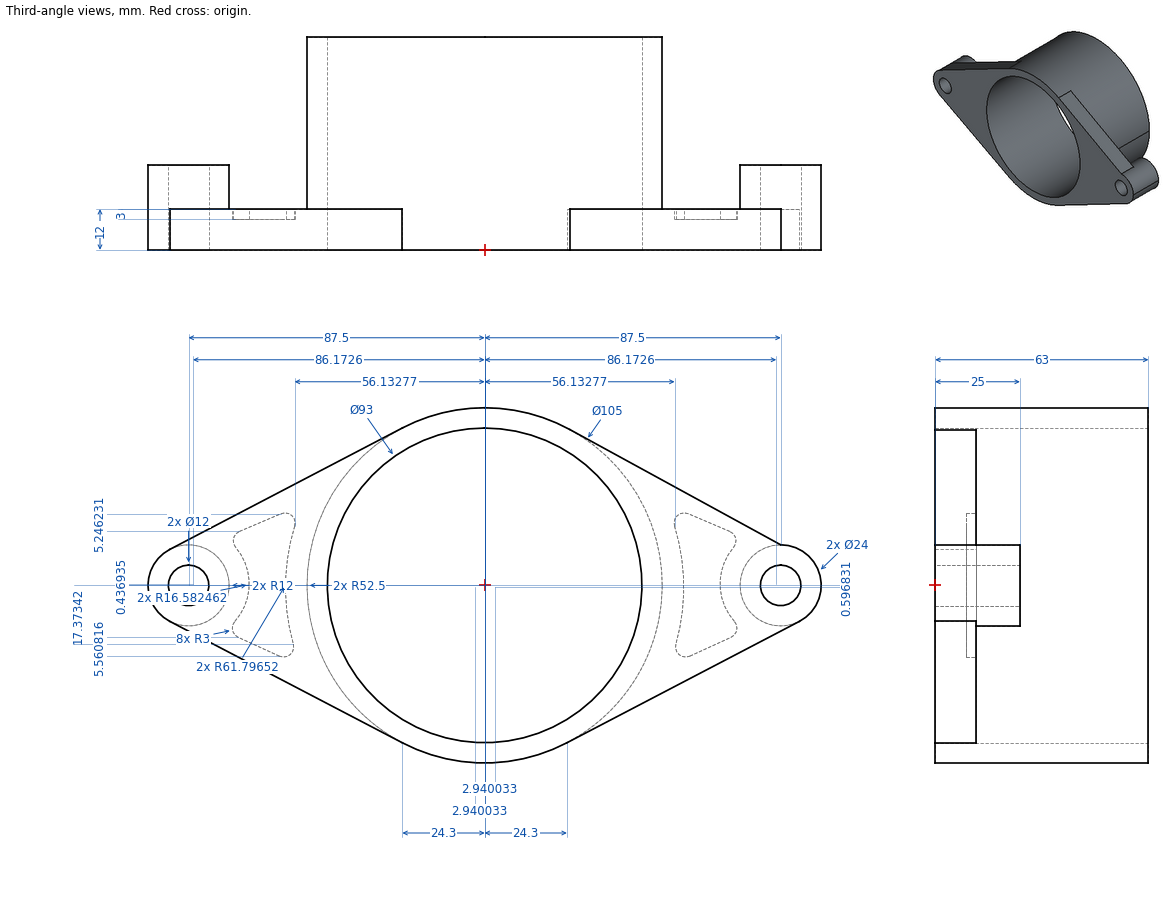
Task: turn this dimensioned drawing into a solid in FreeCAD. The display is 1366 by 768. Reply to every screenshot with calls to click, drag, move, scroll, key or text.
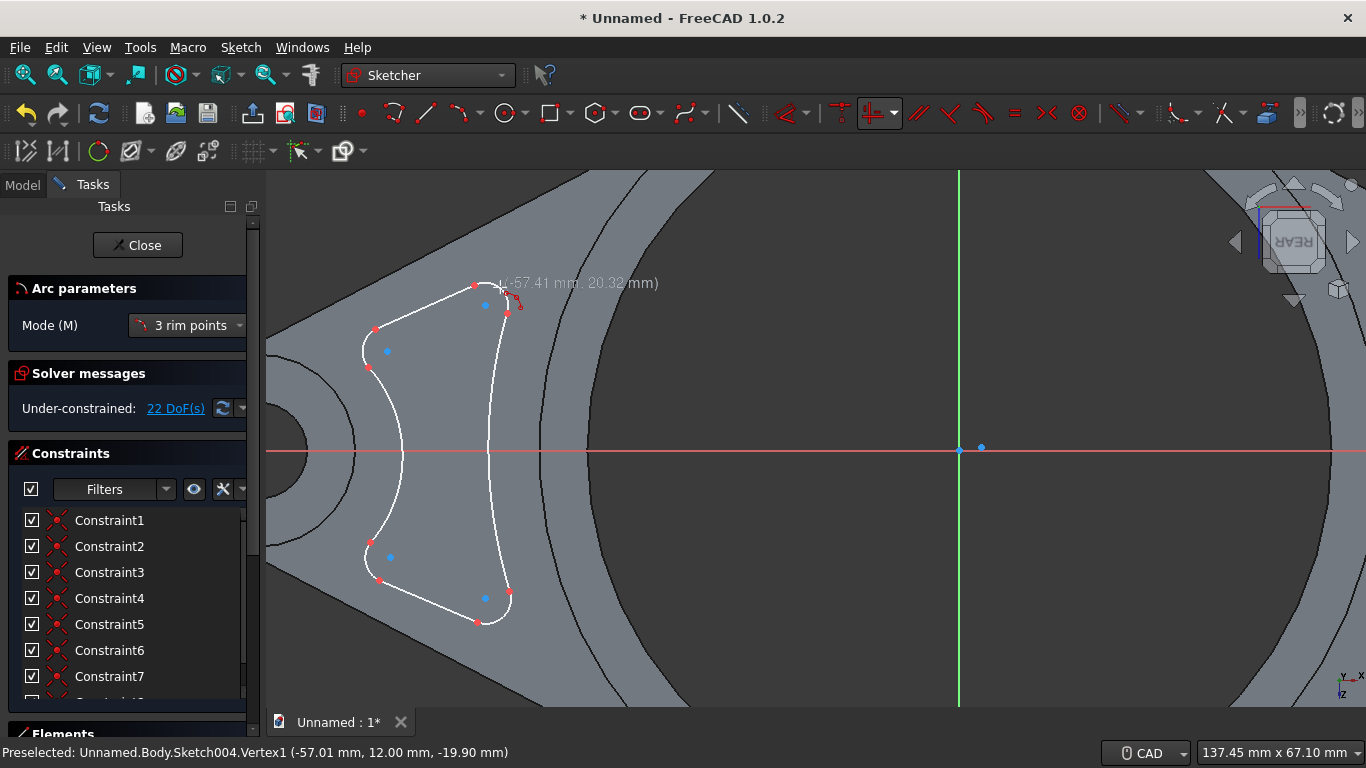
key(g)
key(l)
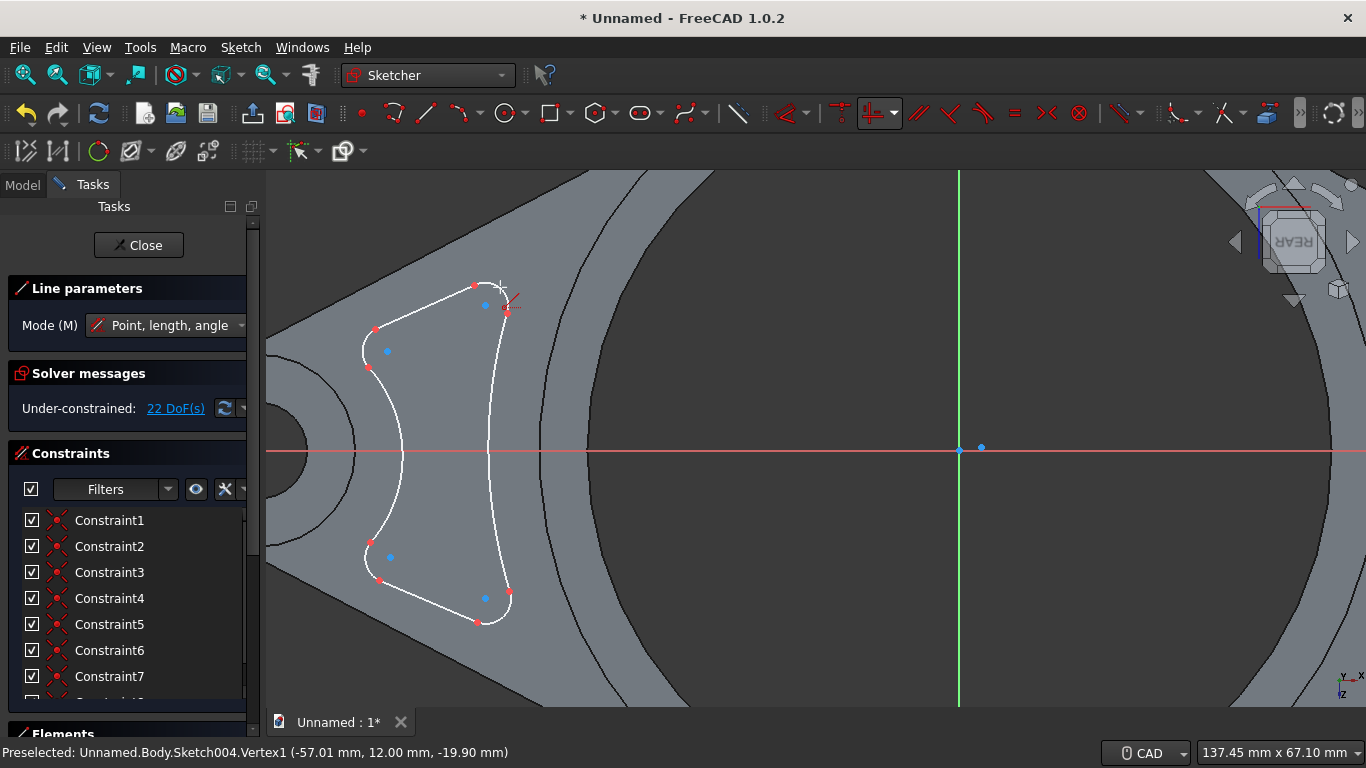
scroll(490, 422, down, 3)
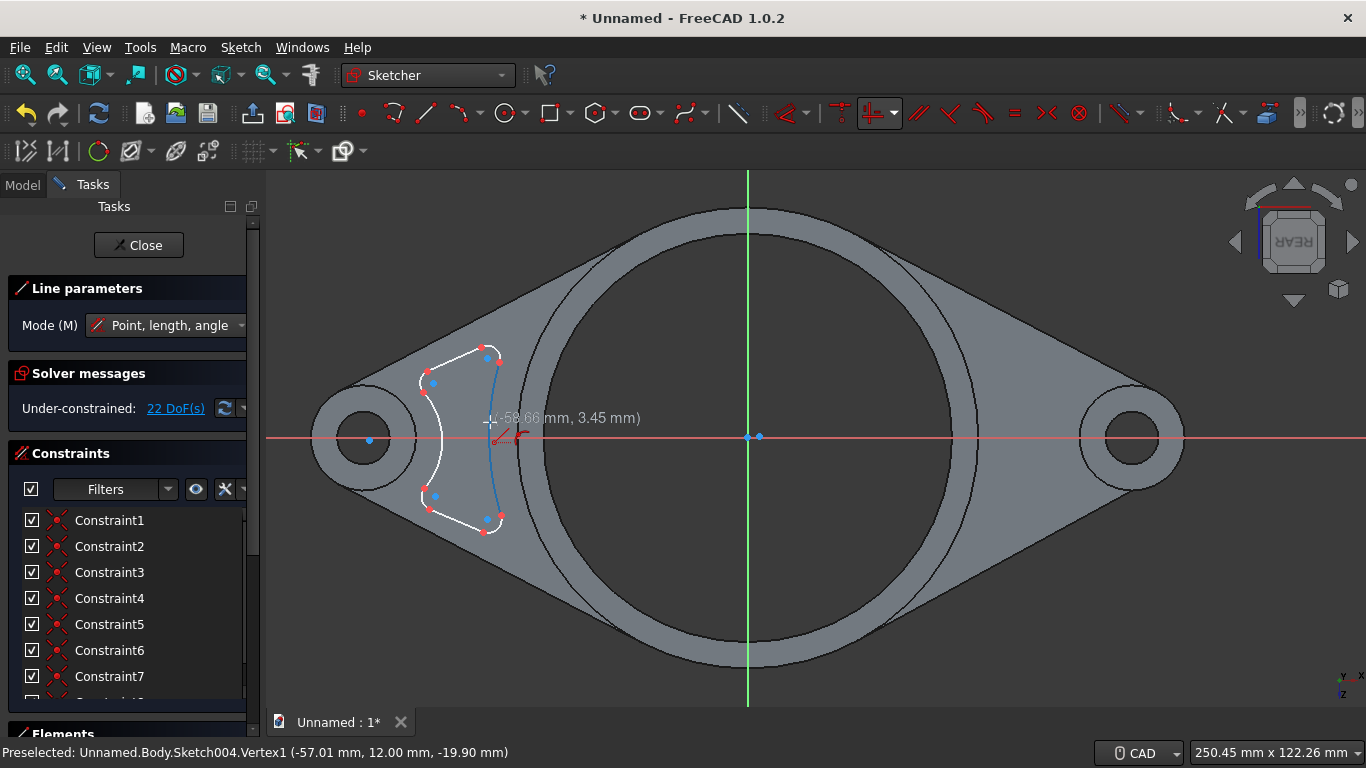
click(1068, 370)
click(1014, 346)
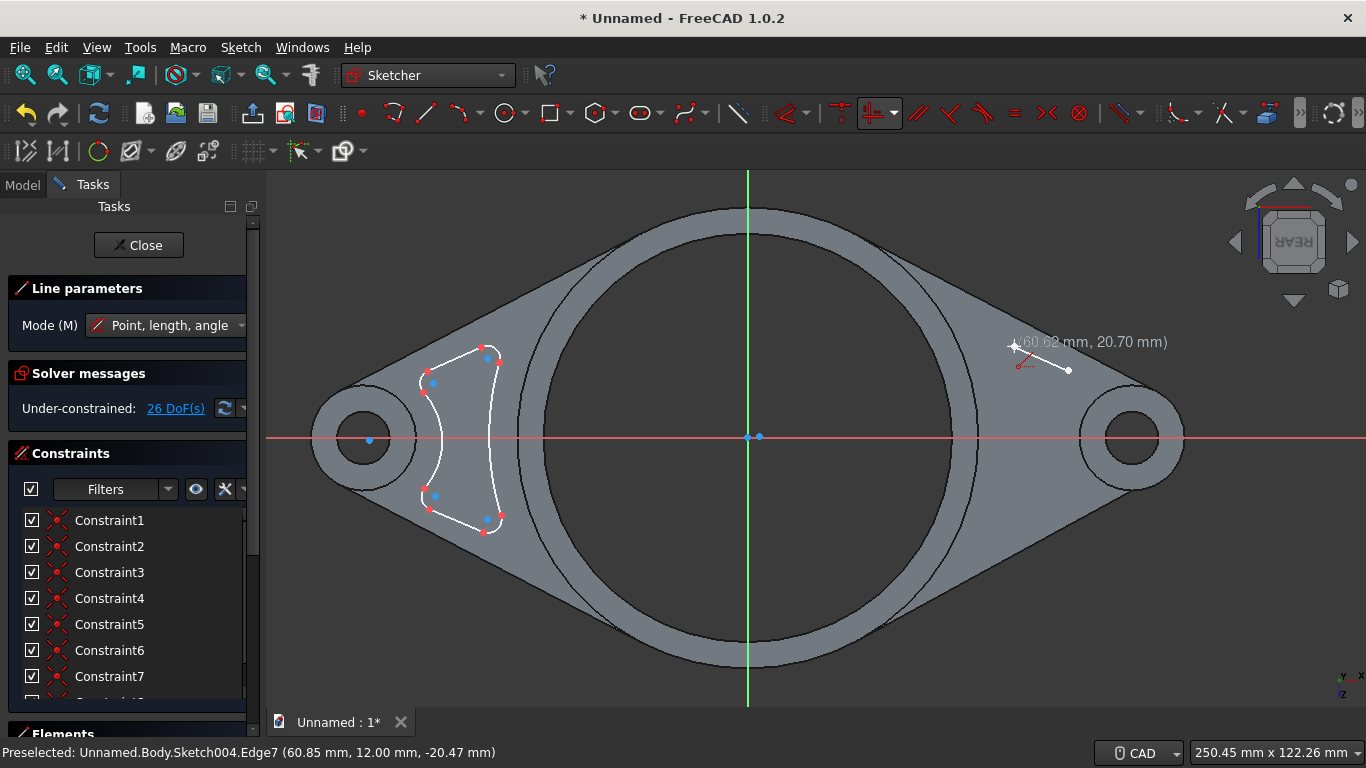
click(1012, 531)
click(1066, 508)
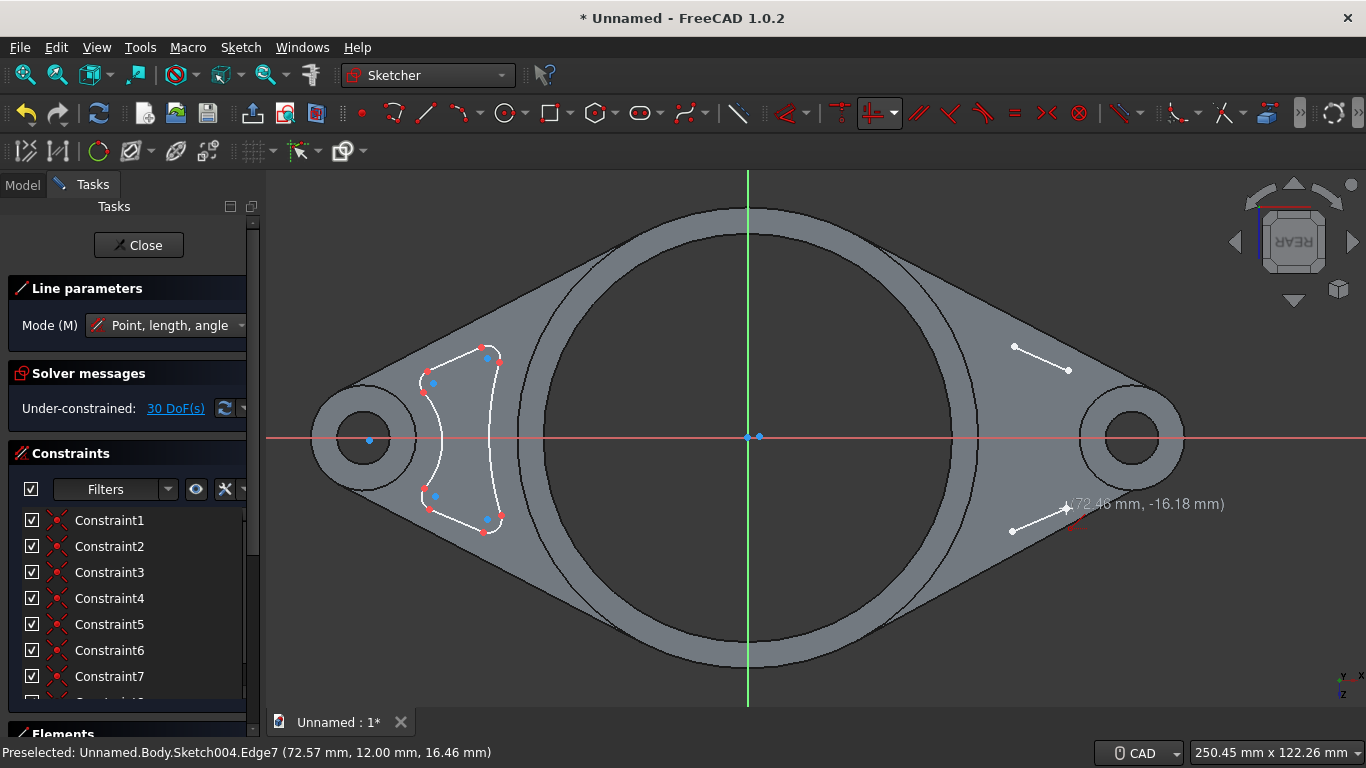
click(460, 114)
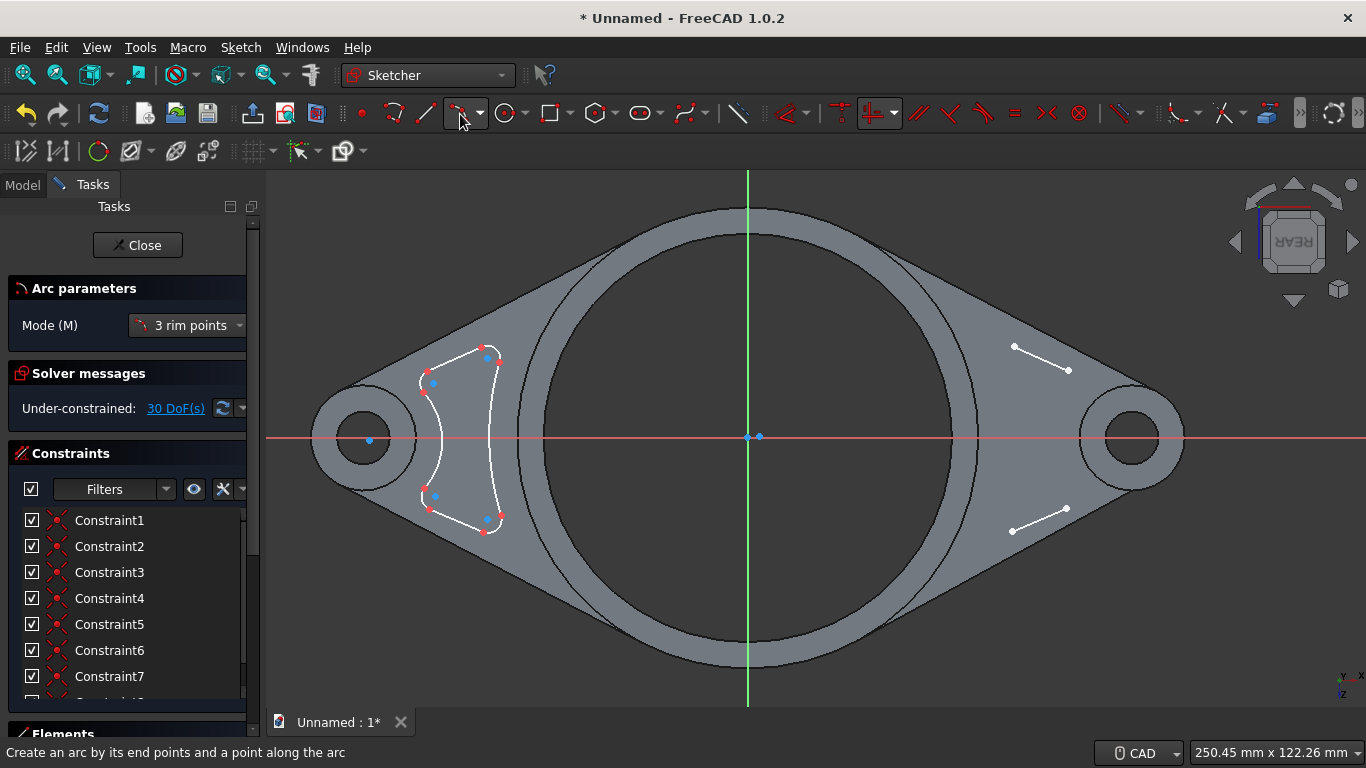
click(1014, 347)
click(996, 362)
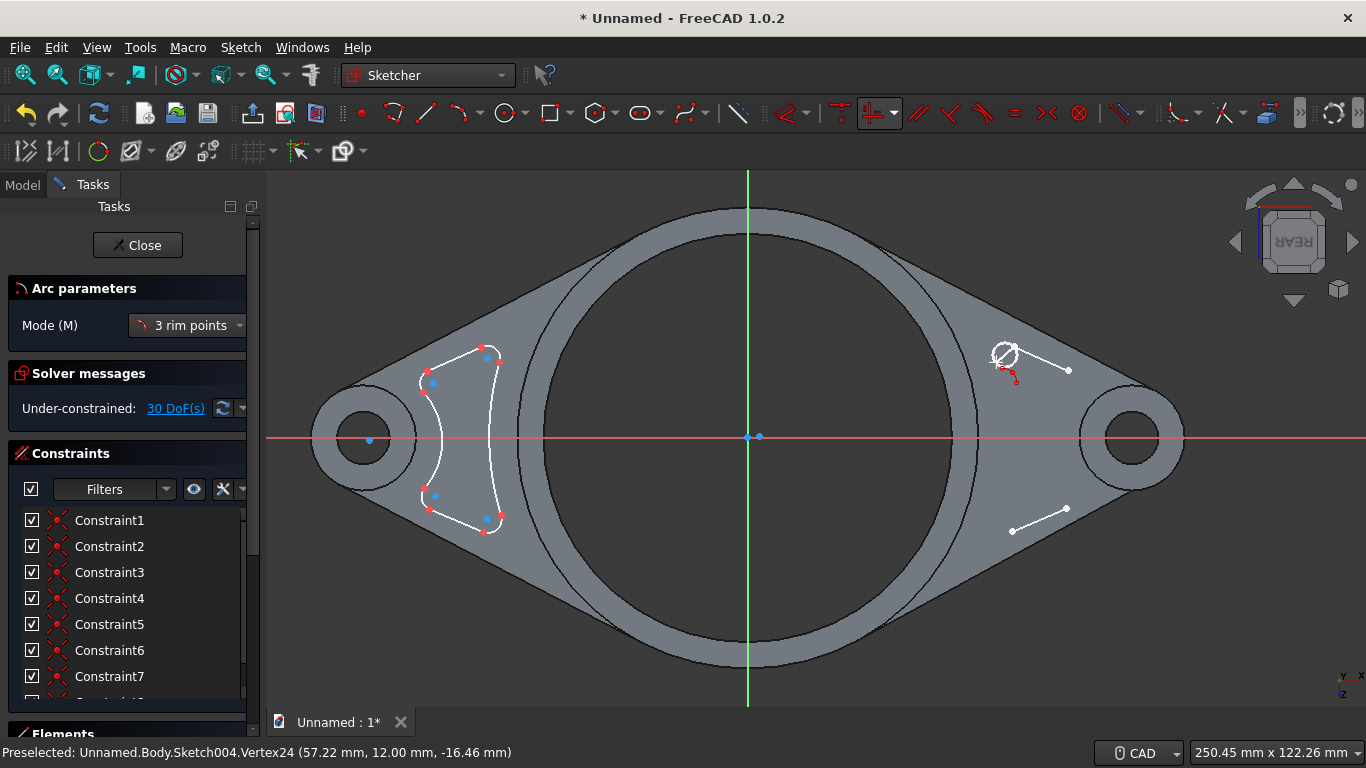
scroll(1000, 348, up, 4)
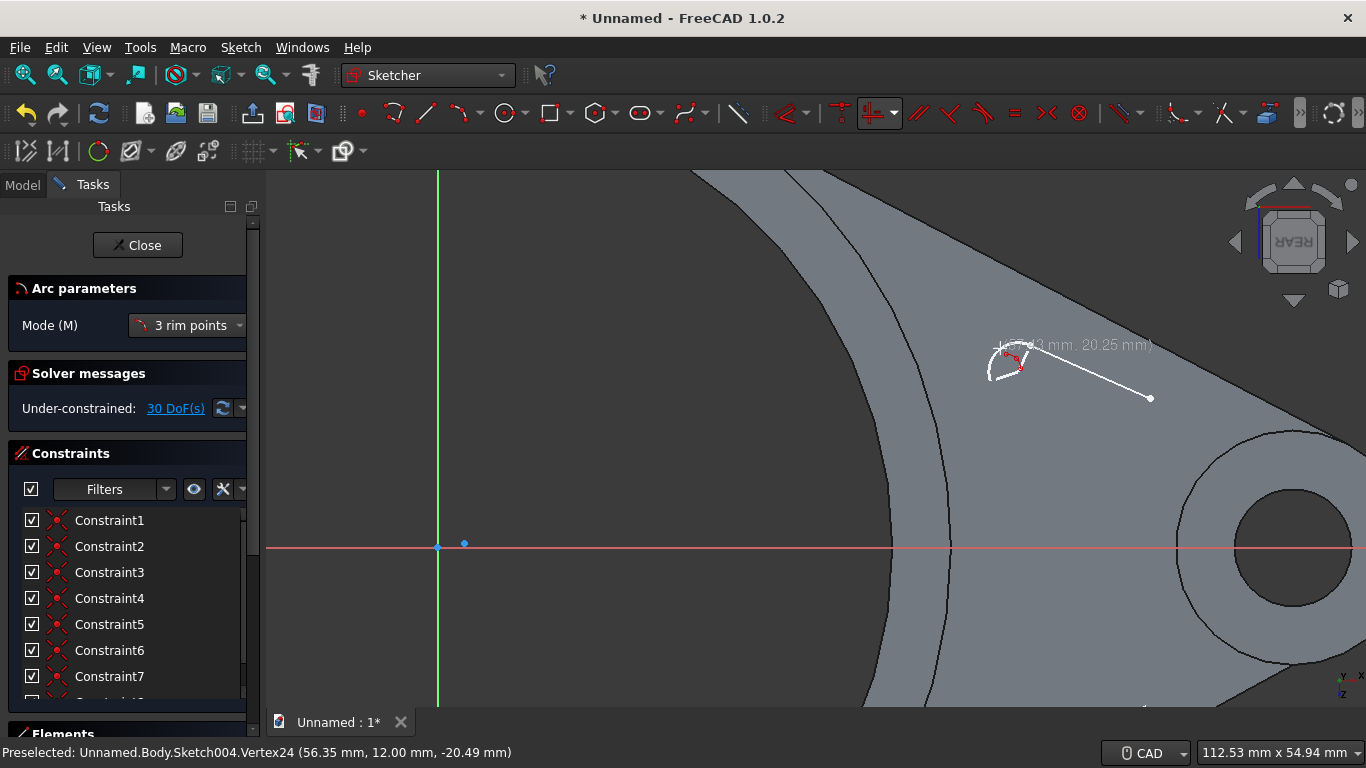
click(1000, 348)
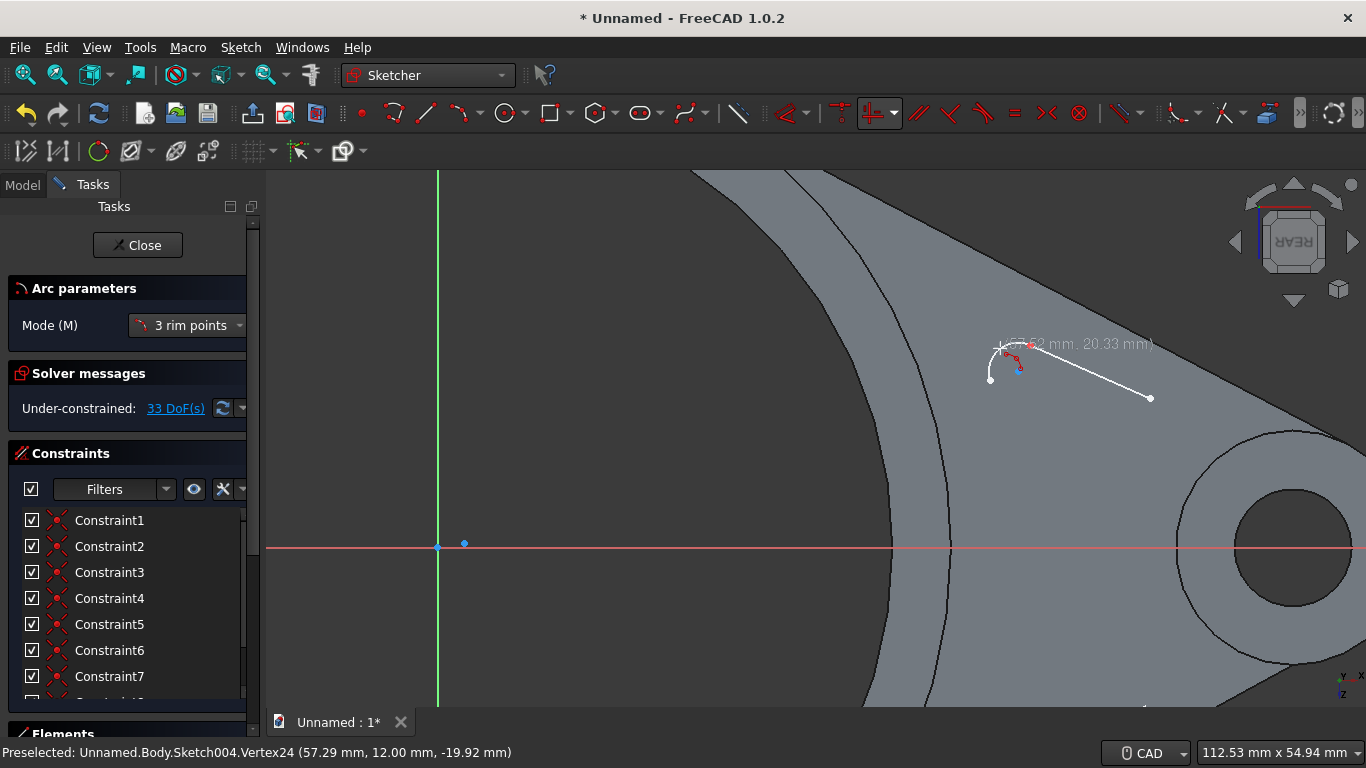
click(990, 381)